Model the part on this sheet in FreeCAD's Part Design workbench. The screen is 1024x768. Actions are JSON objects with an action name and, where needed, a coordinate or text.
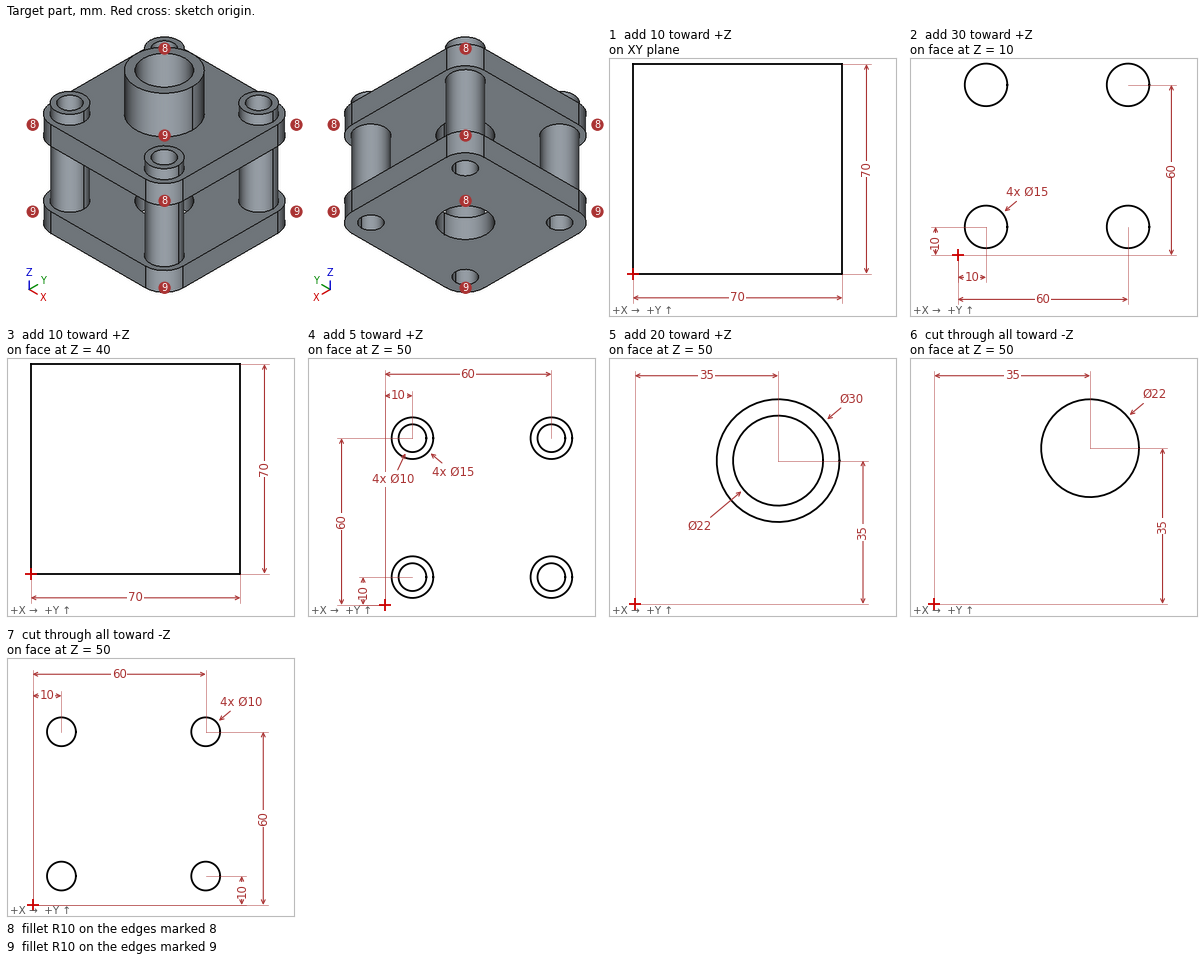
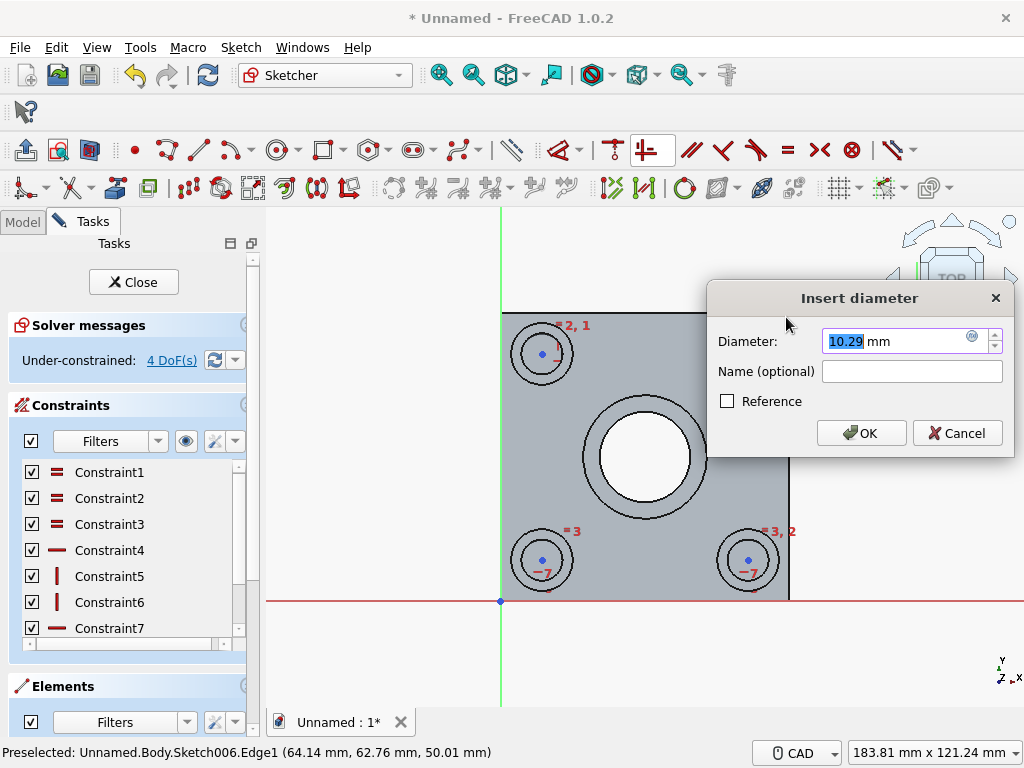
{"action": "type", "text": "10"}
{"action": "key", "text": "Return"}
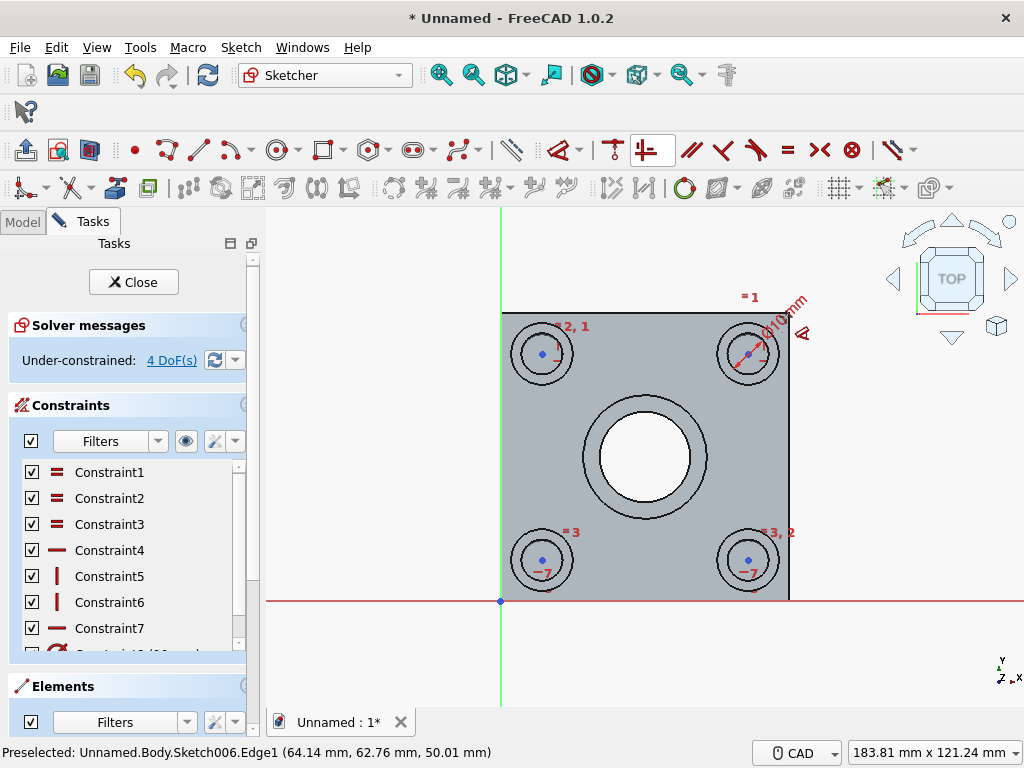
{"action": "left_click", "coordinate": [748, 355]}
{"action": "left_click", "coordinate": [624, 635]}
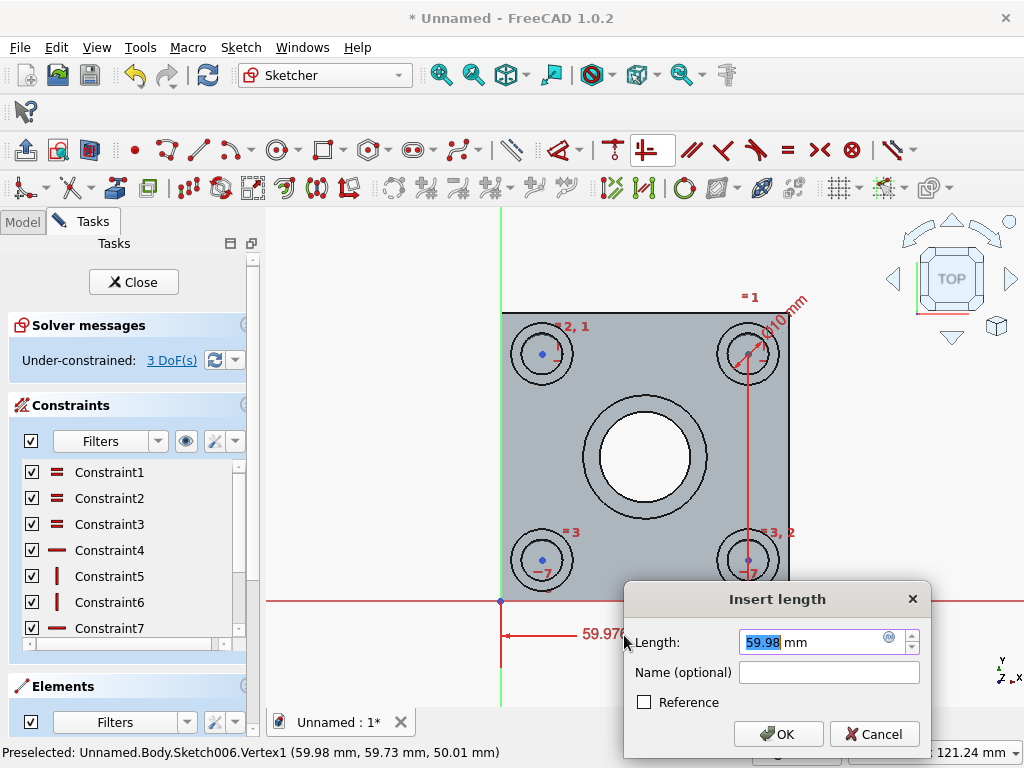
{"action": "type", "text": "60"}
{"action": "key", "text": "Return"}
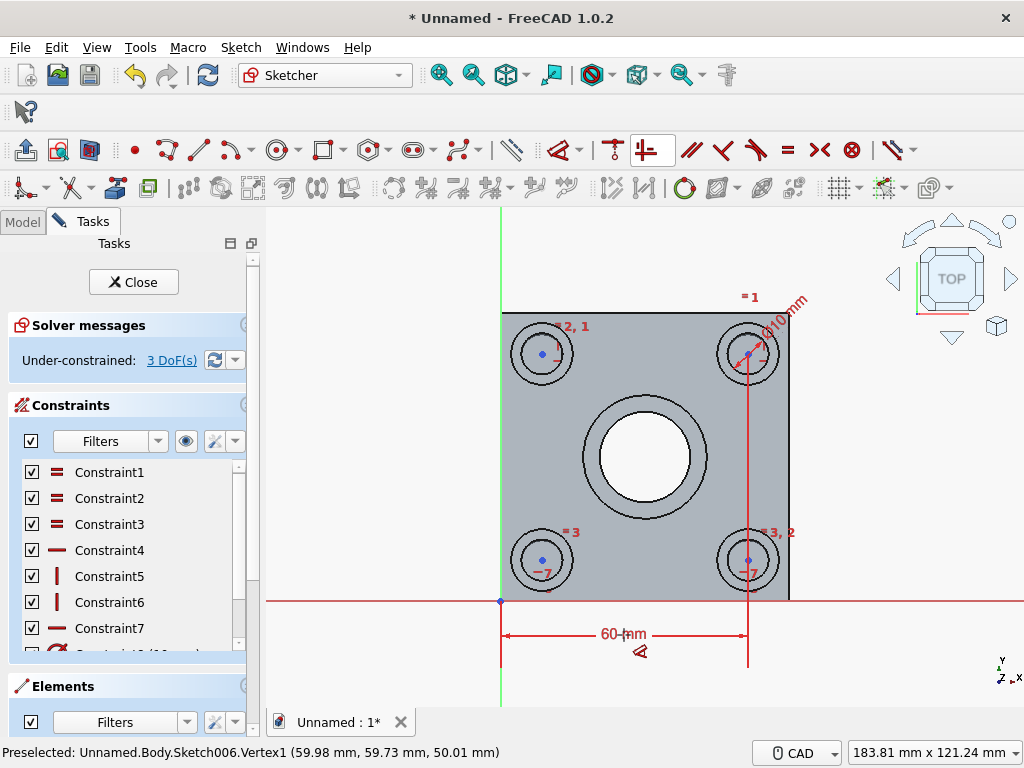
{"action": "left_click", "coordinate": [748, 355]}
{"action": "left_click", "coordinate": [467, 478]}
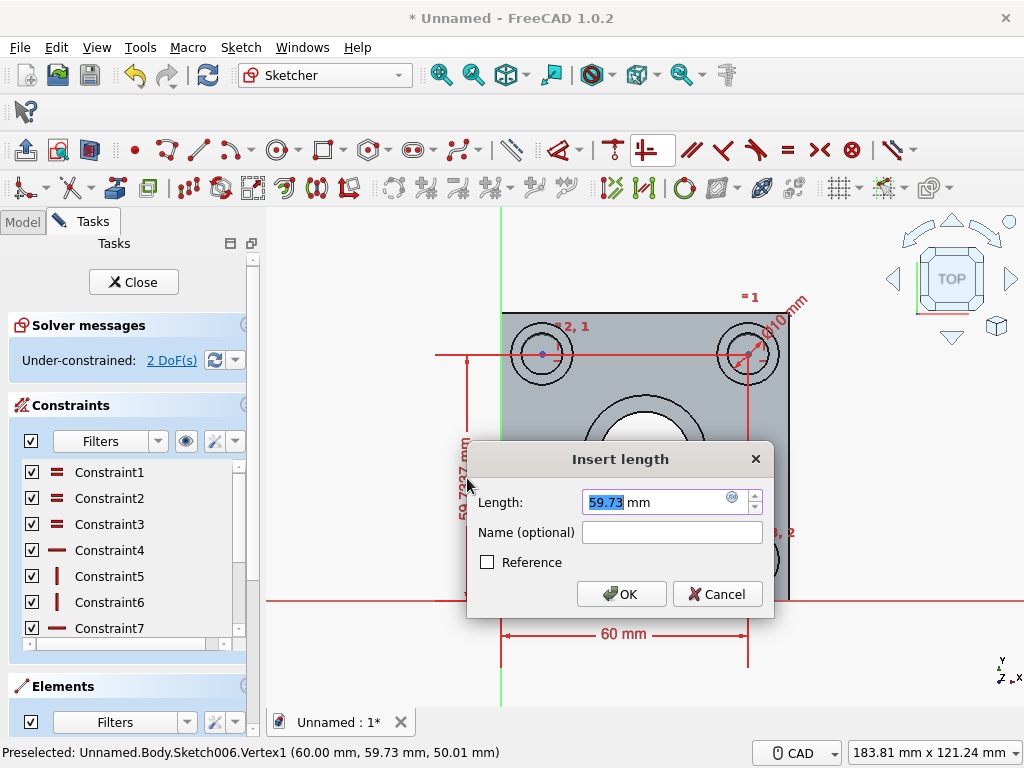
{"action": "type", "text": "60"}
{"action": "key", "text": "Return"}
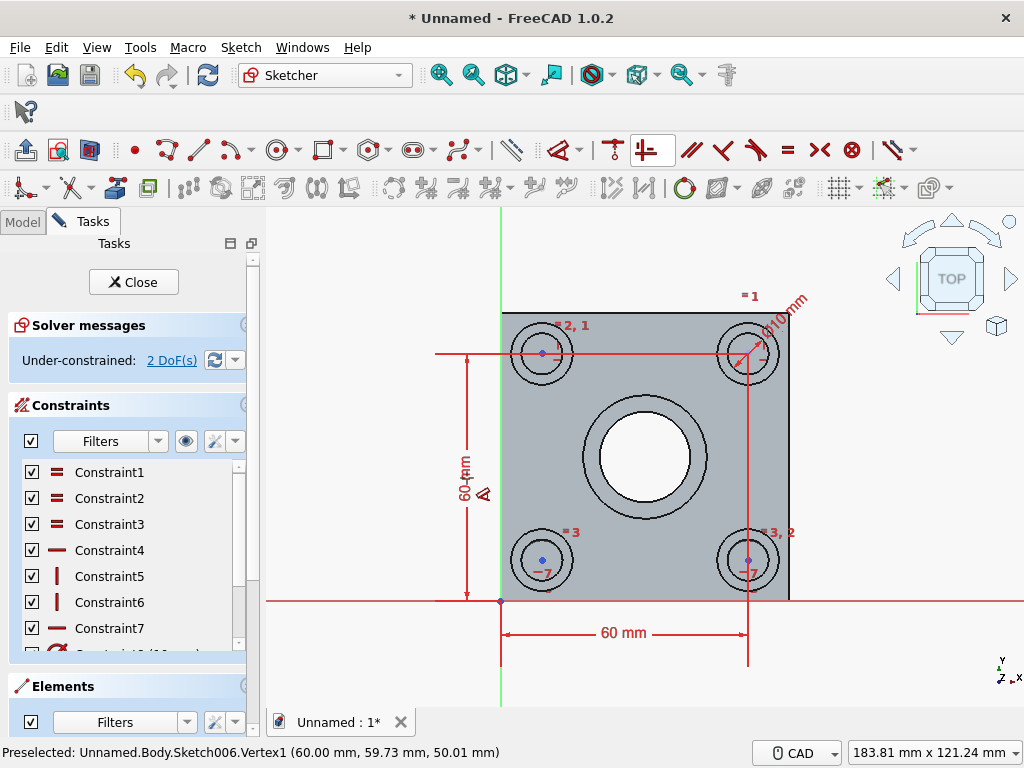
{"action": "left_click", "coordinate": [542, 354]}
{"action": "left_click", "coordinate": [521, 635]}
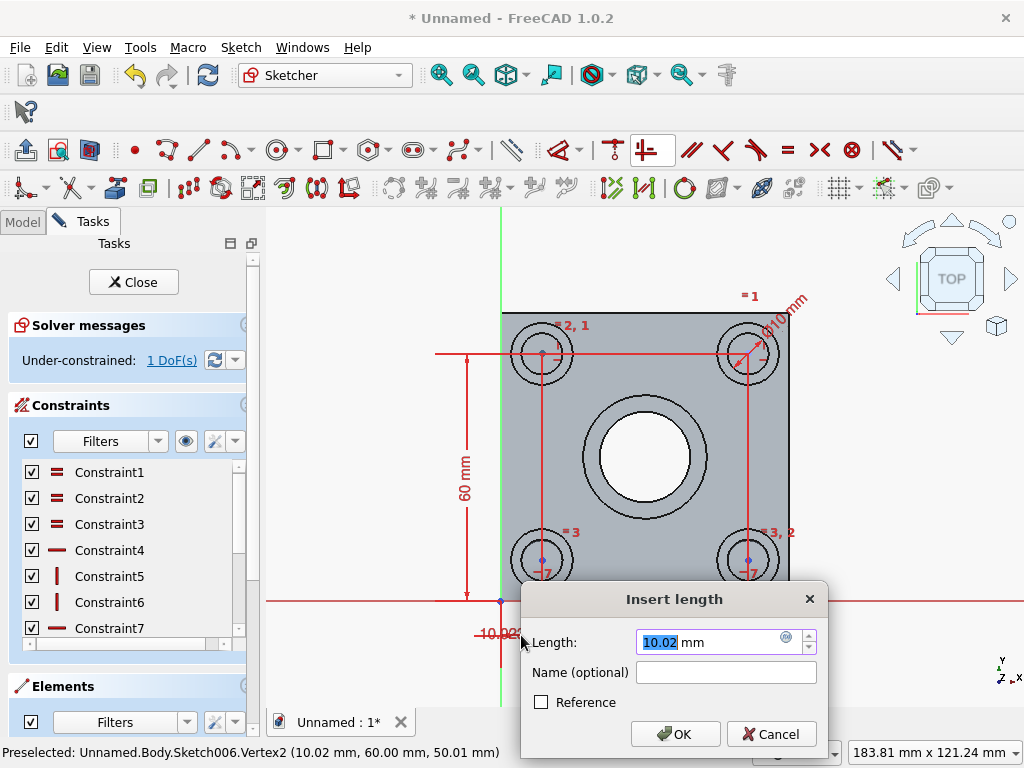
{"action": "type", "text": "10"}
{"action": "key", "text": "Return"}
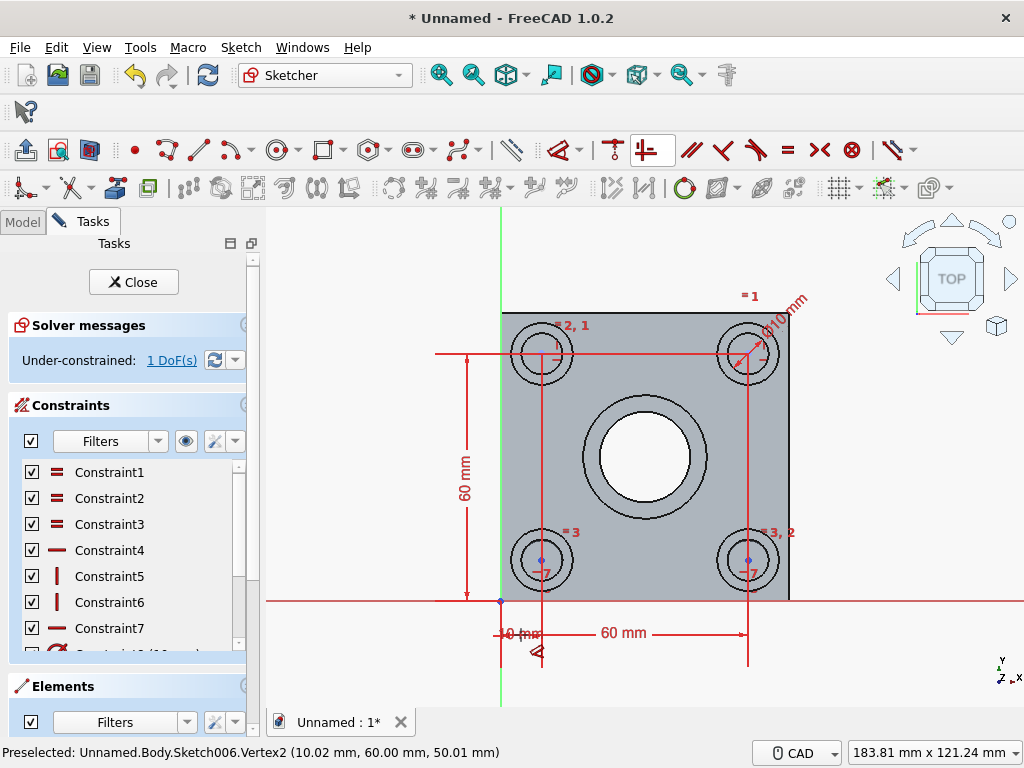
{"action": "left_click", "coordinate": [748, 561]}
{"action": "left_click", "coordinate": [467, 581]}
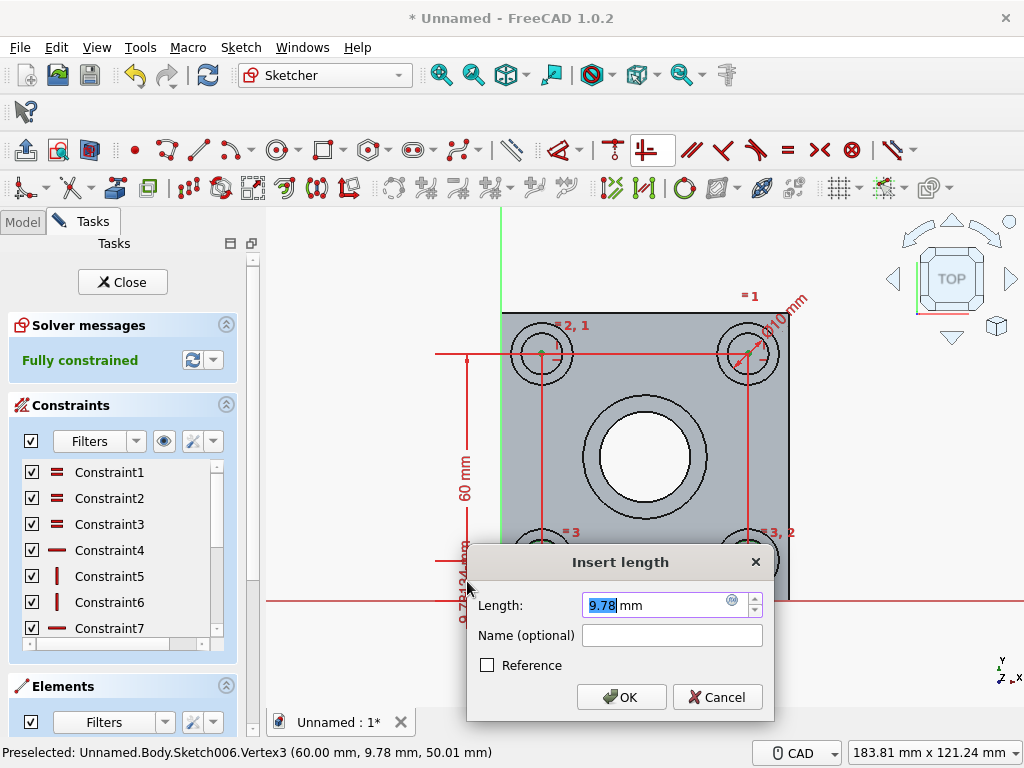
{"action": "type", "text": "10"}
{"action": "key", "text": "Return"}
{"action": "key", "text": "Escape"}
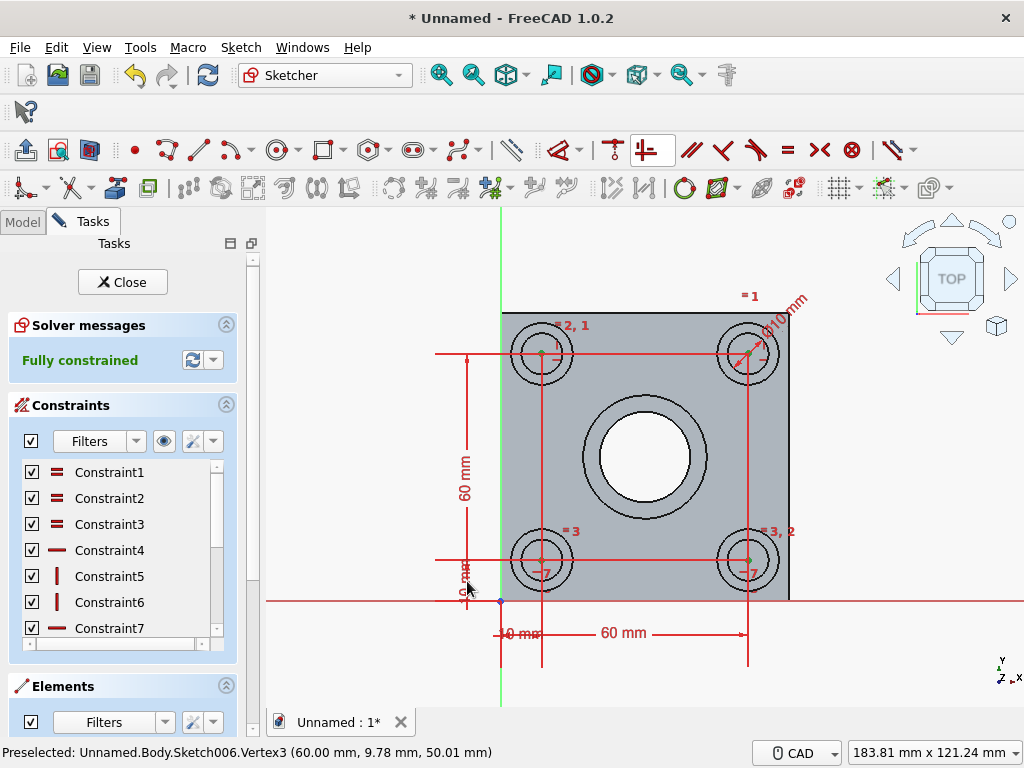
{"action": "left_click", "coordinate": [123, 282]}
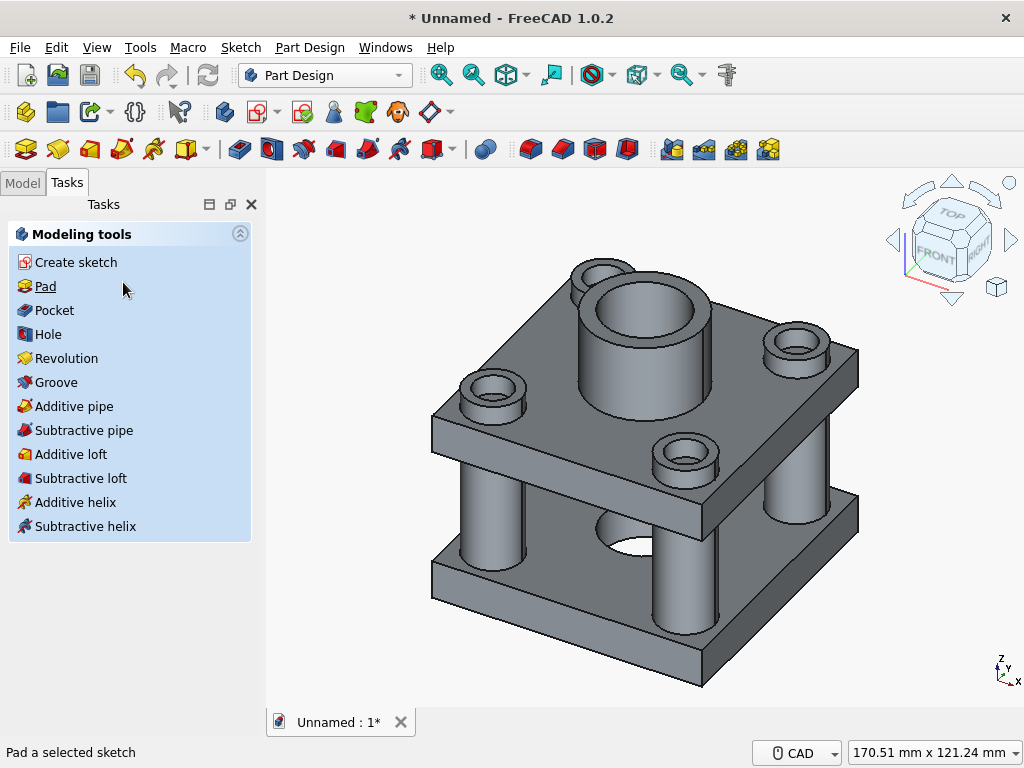
{"action": "left_click", "coordinate": [240, 150]}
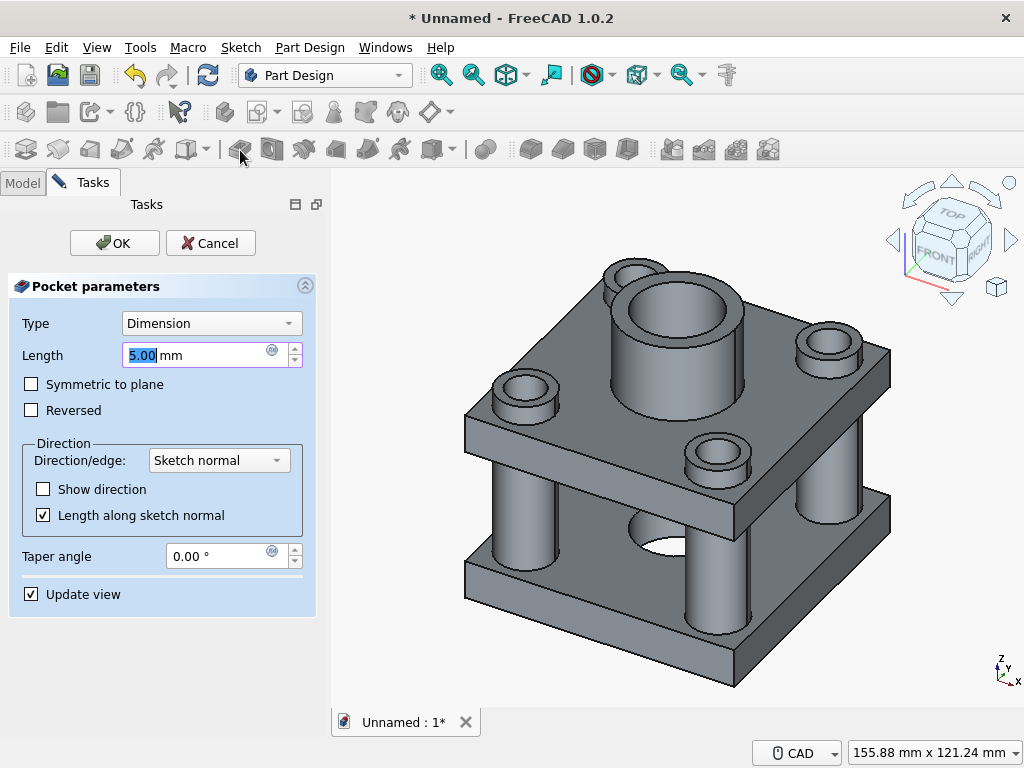
{"action": "left_click", "coordinate": [212, 324]}